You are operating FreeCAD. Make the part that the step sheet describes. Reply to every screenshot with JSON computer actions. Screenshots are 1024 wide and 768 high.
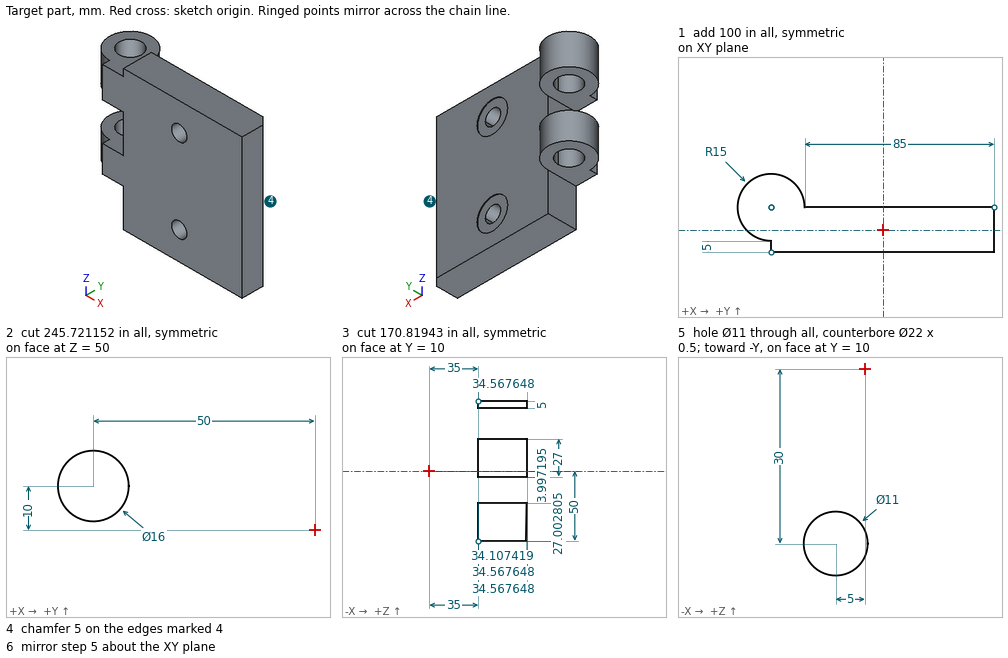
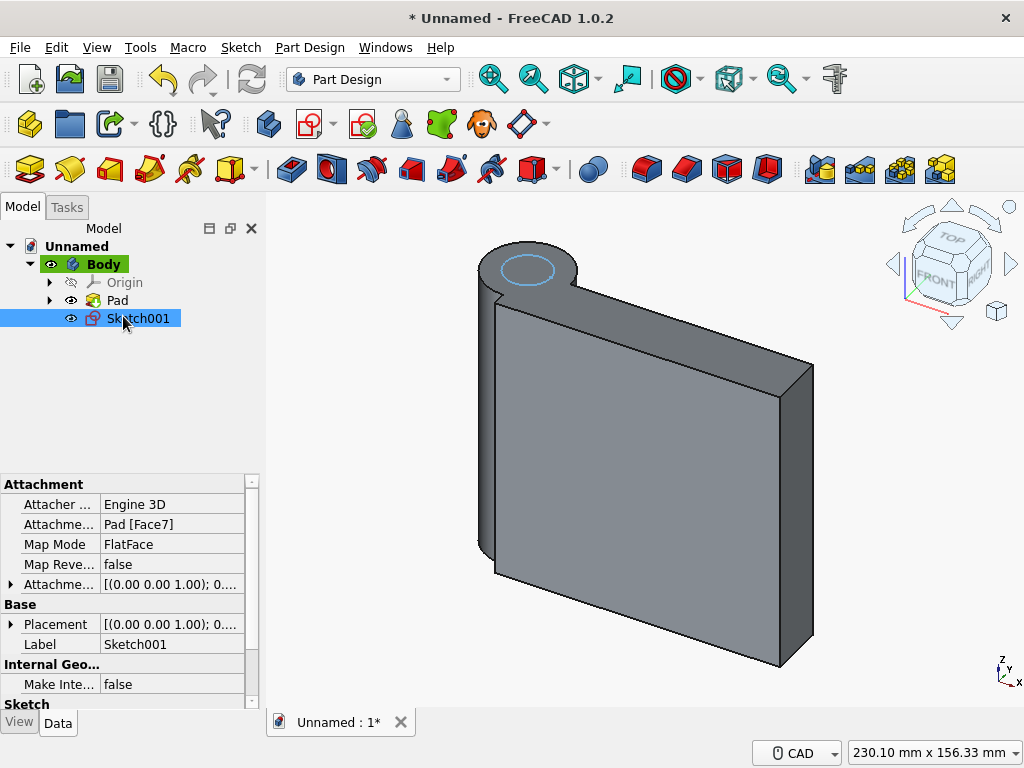
{"action": "left_click", "coordinate": [292, 170]}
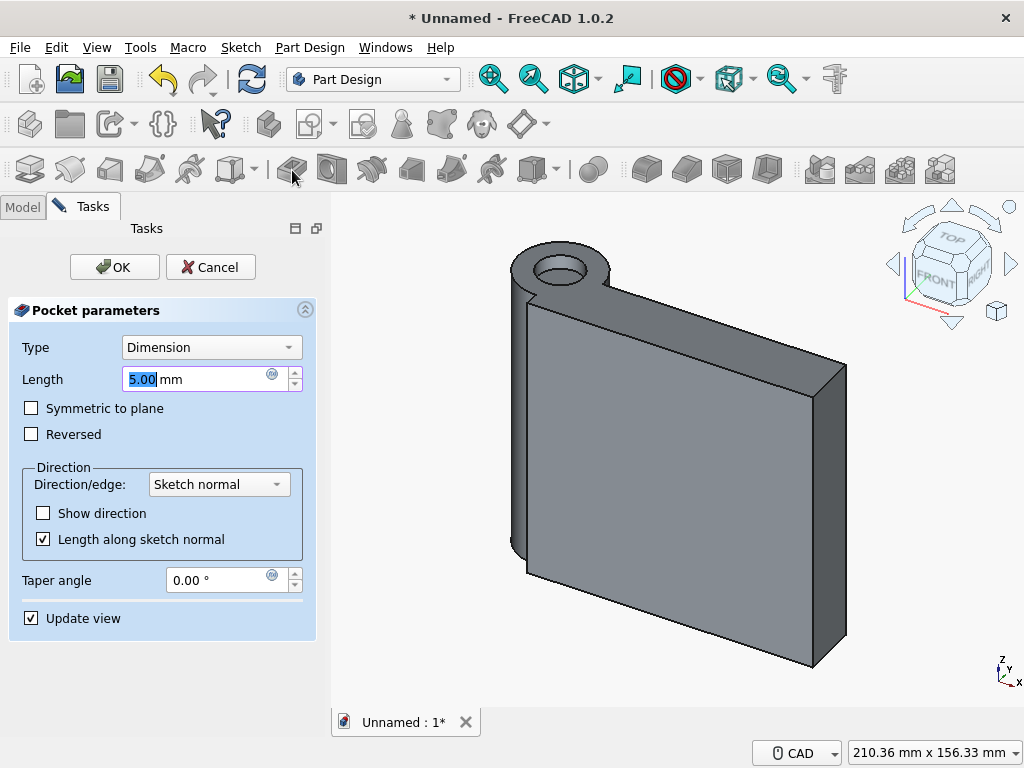
{"action": "type", "text": "245.721152"}
{"action": "key", "text": "Tab"}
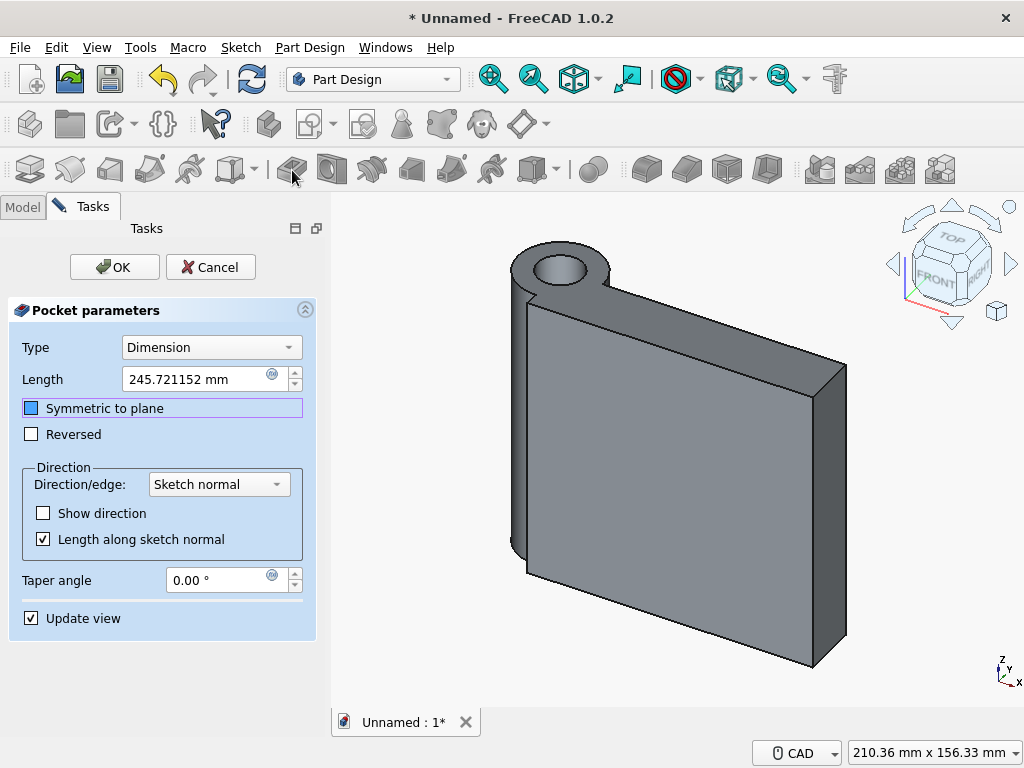
{"action": "left_click", "coordinate": [30, 408]}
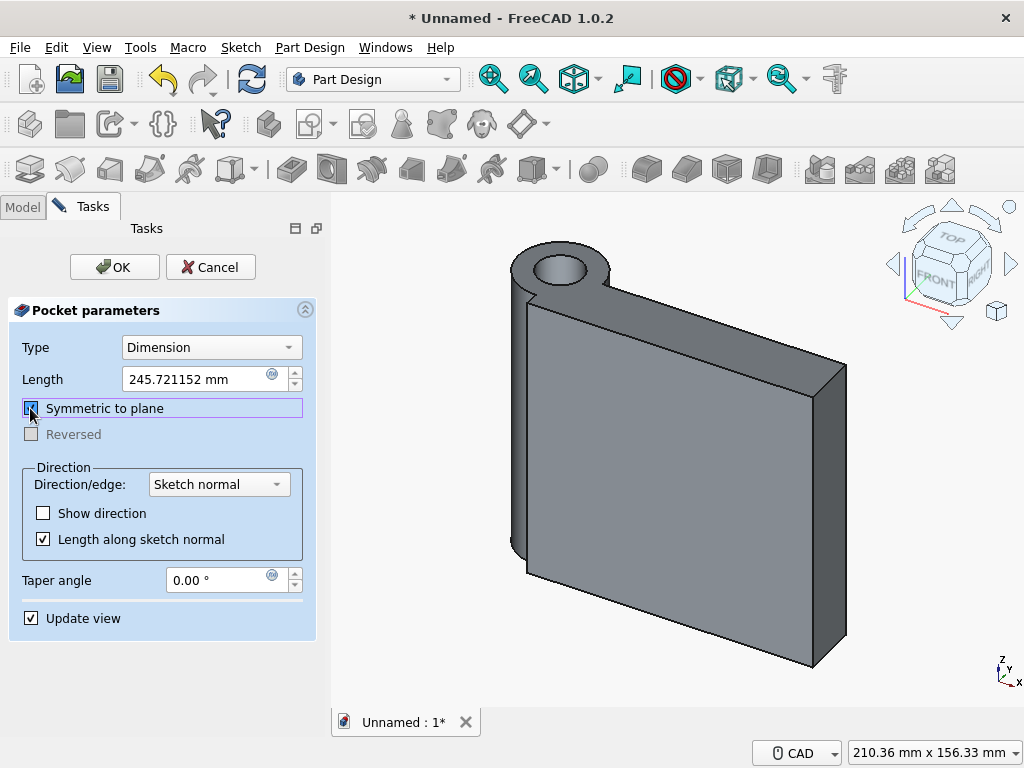
{"action": "left_click", "coordinate": [115, 267]}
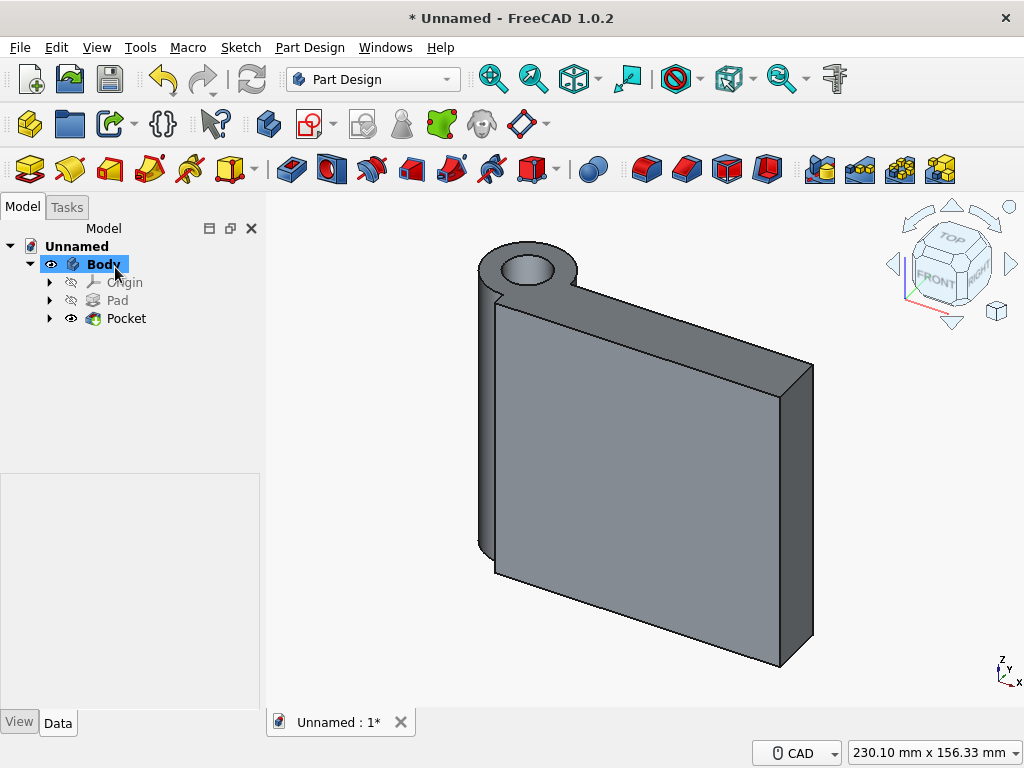
{"action": "key", "text": "4"}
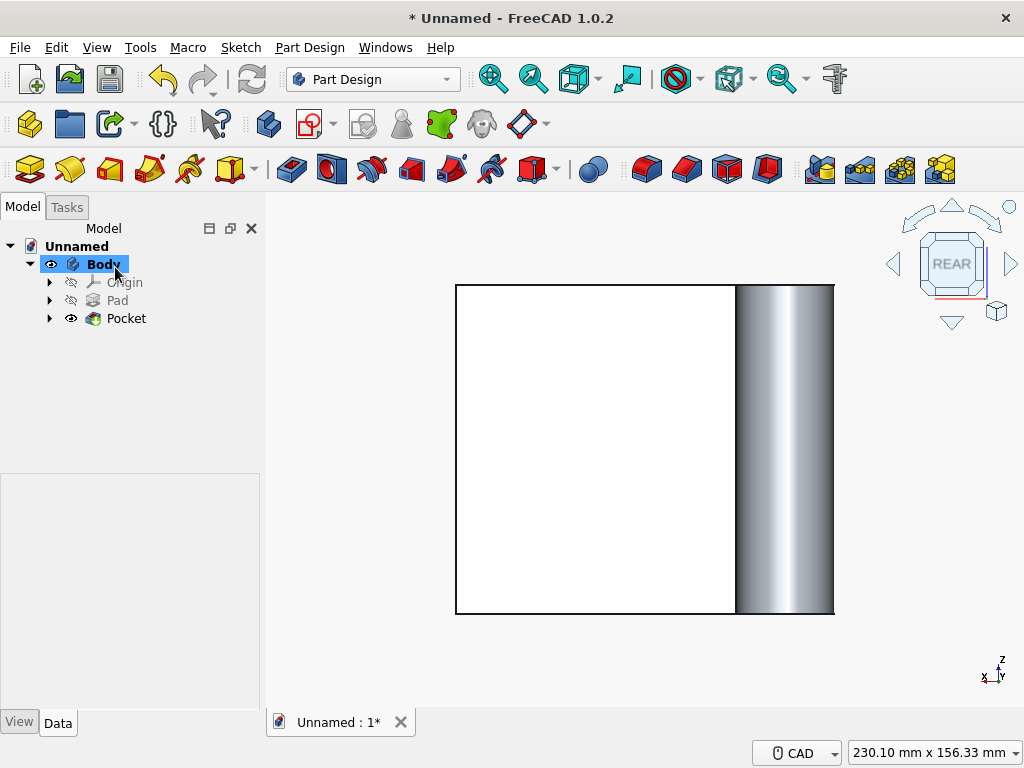
{"action": "left_click", "coordinate": [596, 448]}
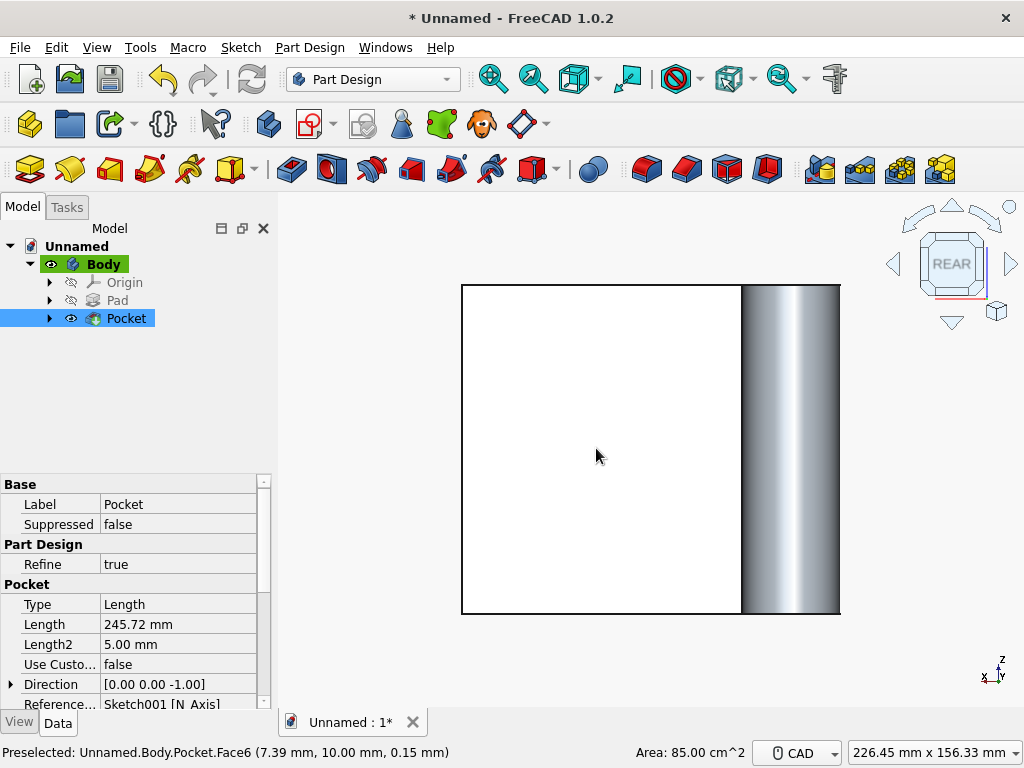
{"action": "left_click", "coordinate": [310, 124]}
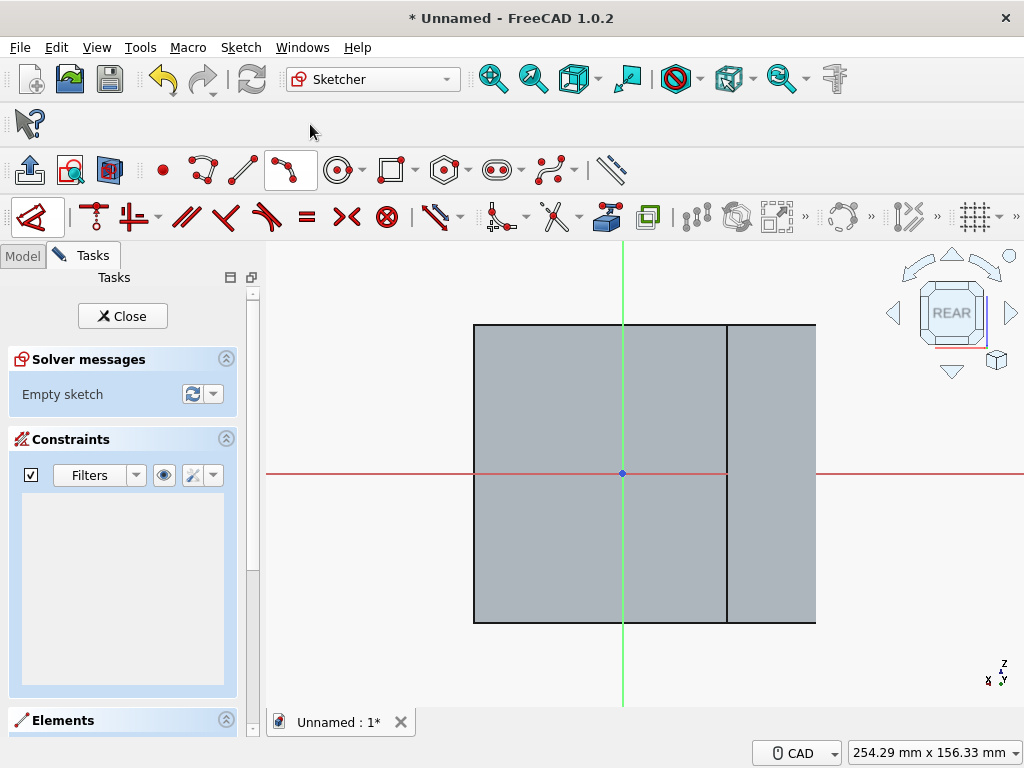
{"action": "left_click", "coordinate": [204, 170]}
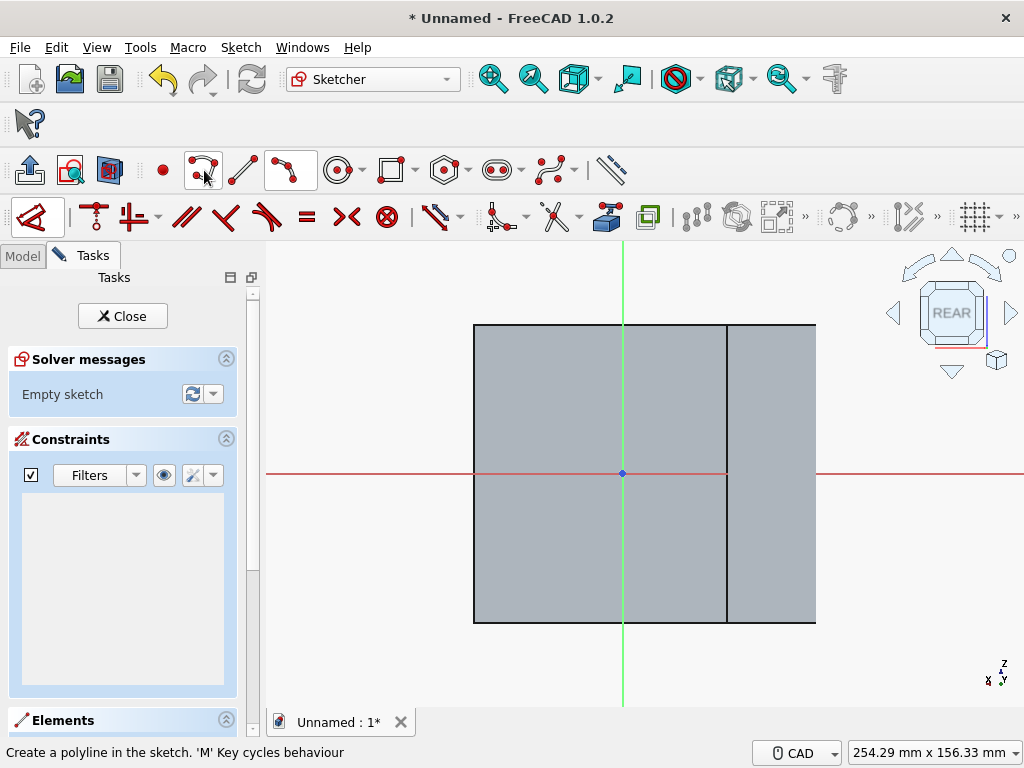
{"action": "left_click", "coordinate": [727, 543]}
{"action": "left_click", "coordinate": [727, 623]}
{"action": "left_click", "coordinate": [829, 623]}
{"action": "left_click", "coordinate": [834, 543]}
{"action": "left_click", "coordinate": [727, 544]}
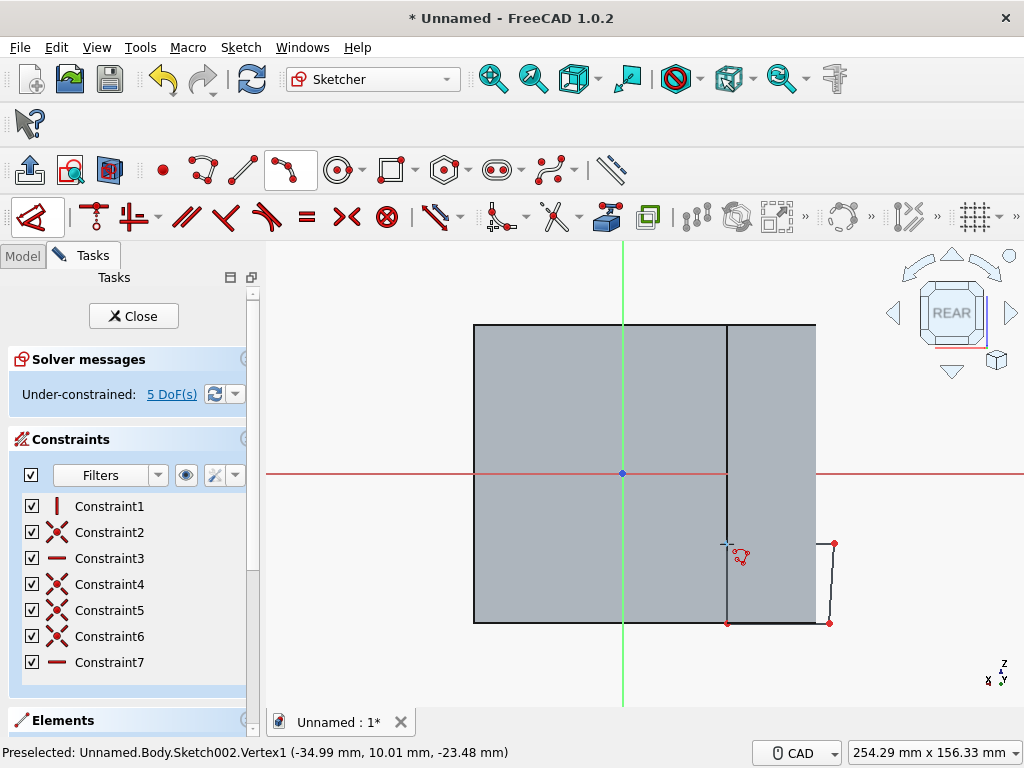
{"action": "left_click", "coordinate": [392, 170]}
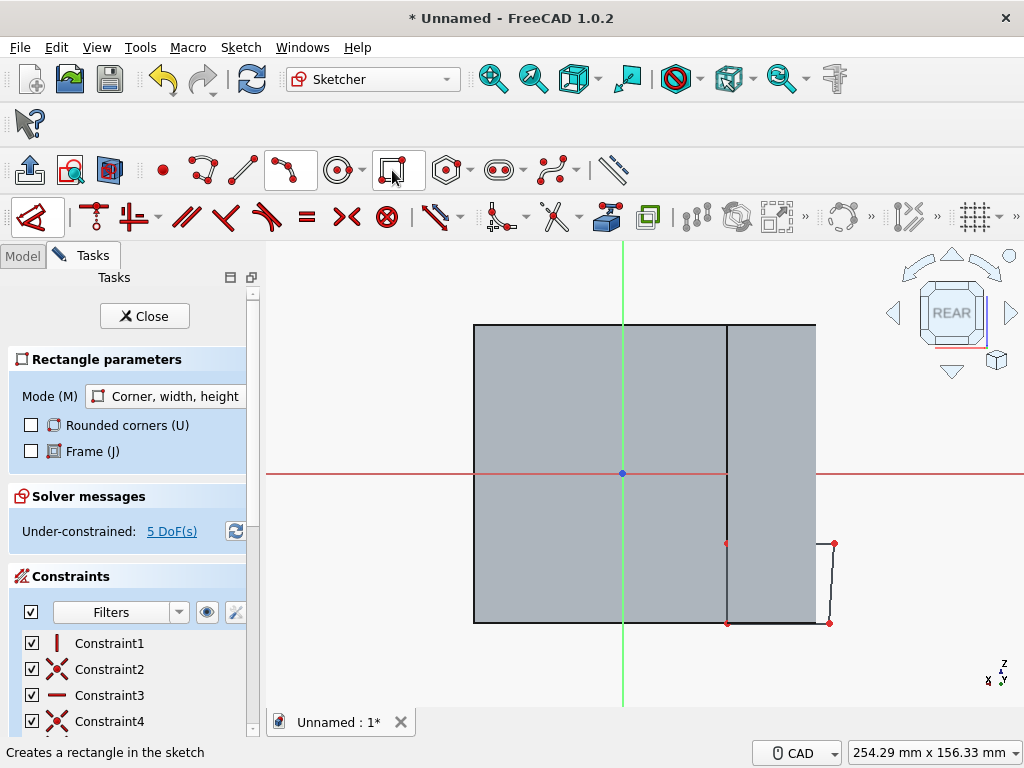
{"action": "left_click", "coordinate": [727, 405]}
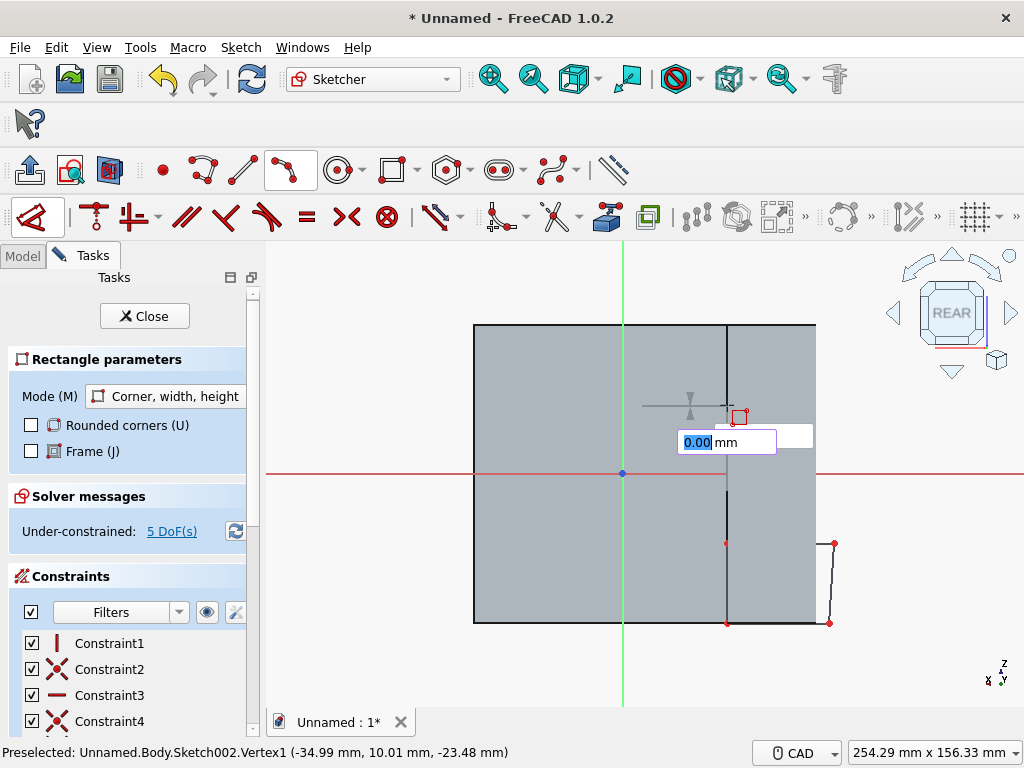
{"action": "scroll", "coordinate": [830, 486], "scroll_direction": "up", "scroll_amount": 2}
{"action": "mouse_move", "coordinate": [830, 486]}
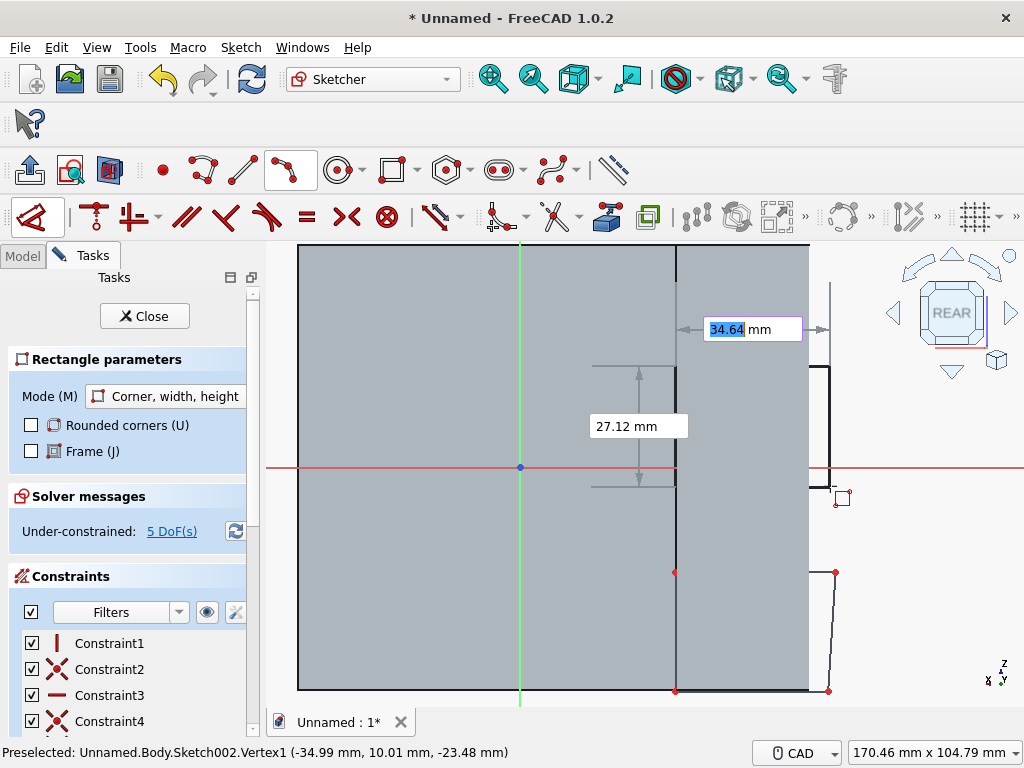
{"action": "type", "text": "34.567648"}
{"action": "key", "text": "Tab"}
{"action": "type", "text": "27"}
{"action": "key", "text": "Return"}